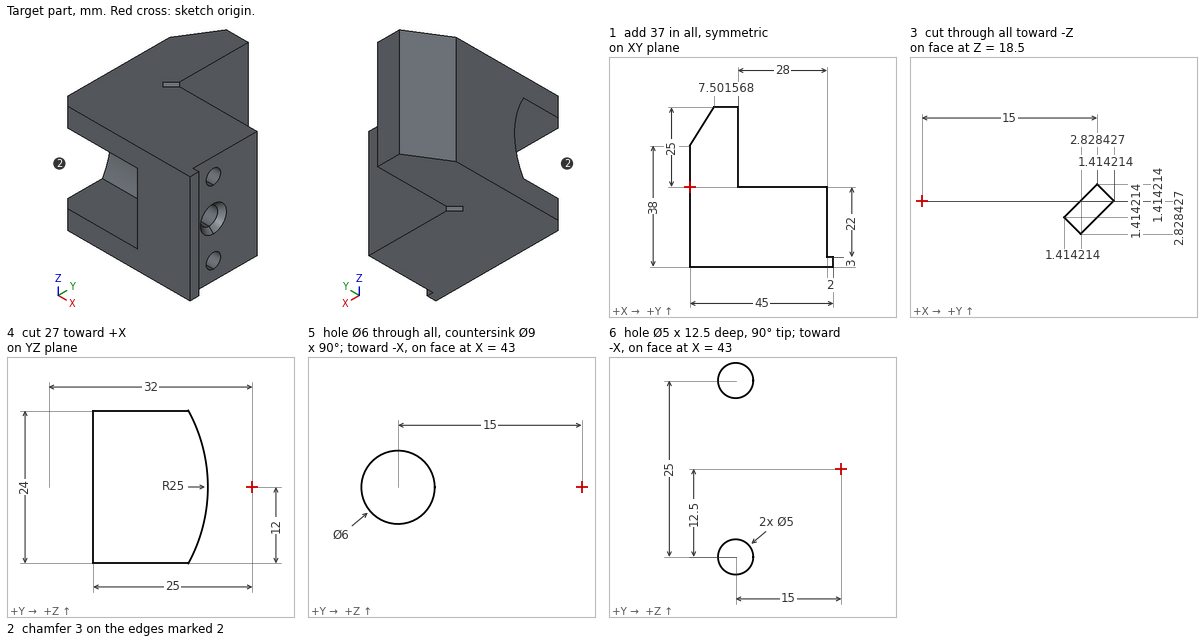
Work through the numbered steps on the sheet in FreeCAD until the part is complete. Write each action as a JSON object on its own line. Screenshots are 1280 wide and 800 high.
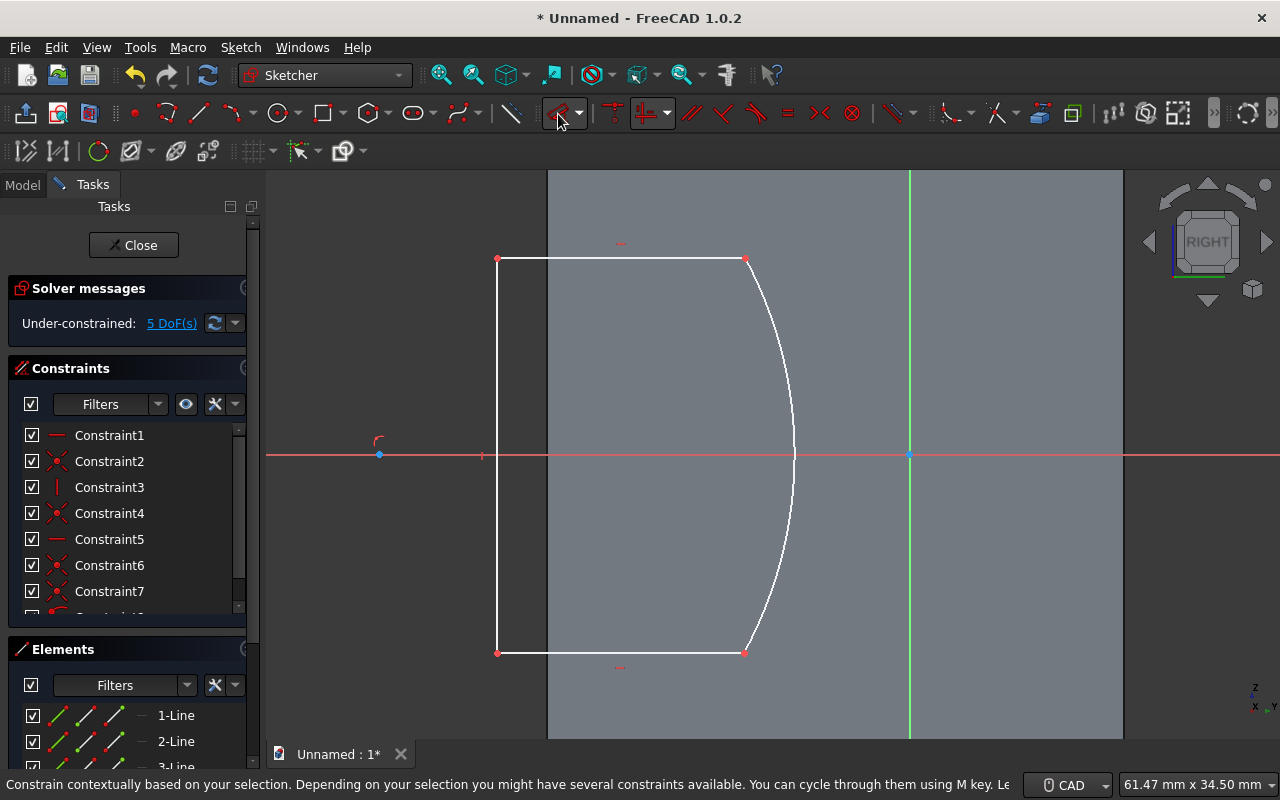
{"action": "left_click", "coordinate": [786, 537]}
{"action": "left_click", "coordinate": [817, 543]}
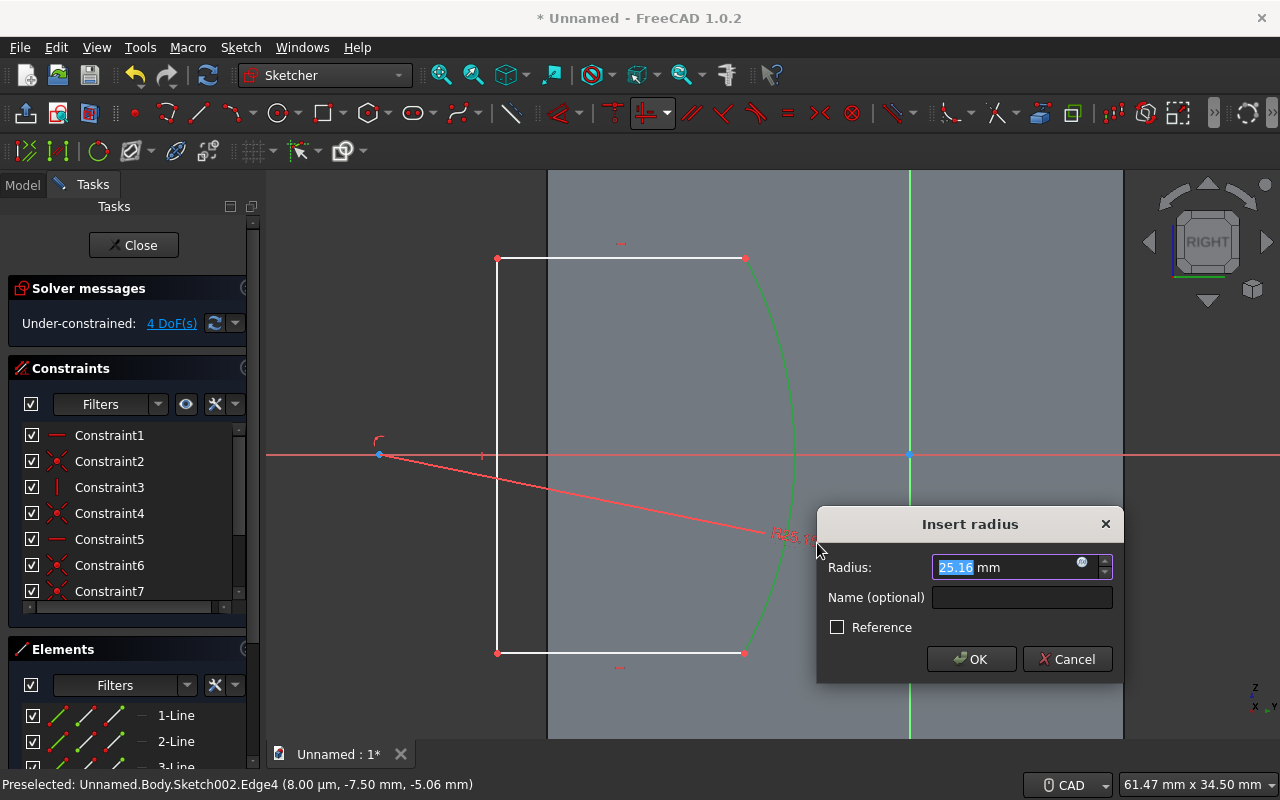
{"action": "type", "text": "25"}
{"action": "key", "text": "Return"}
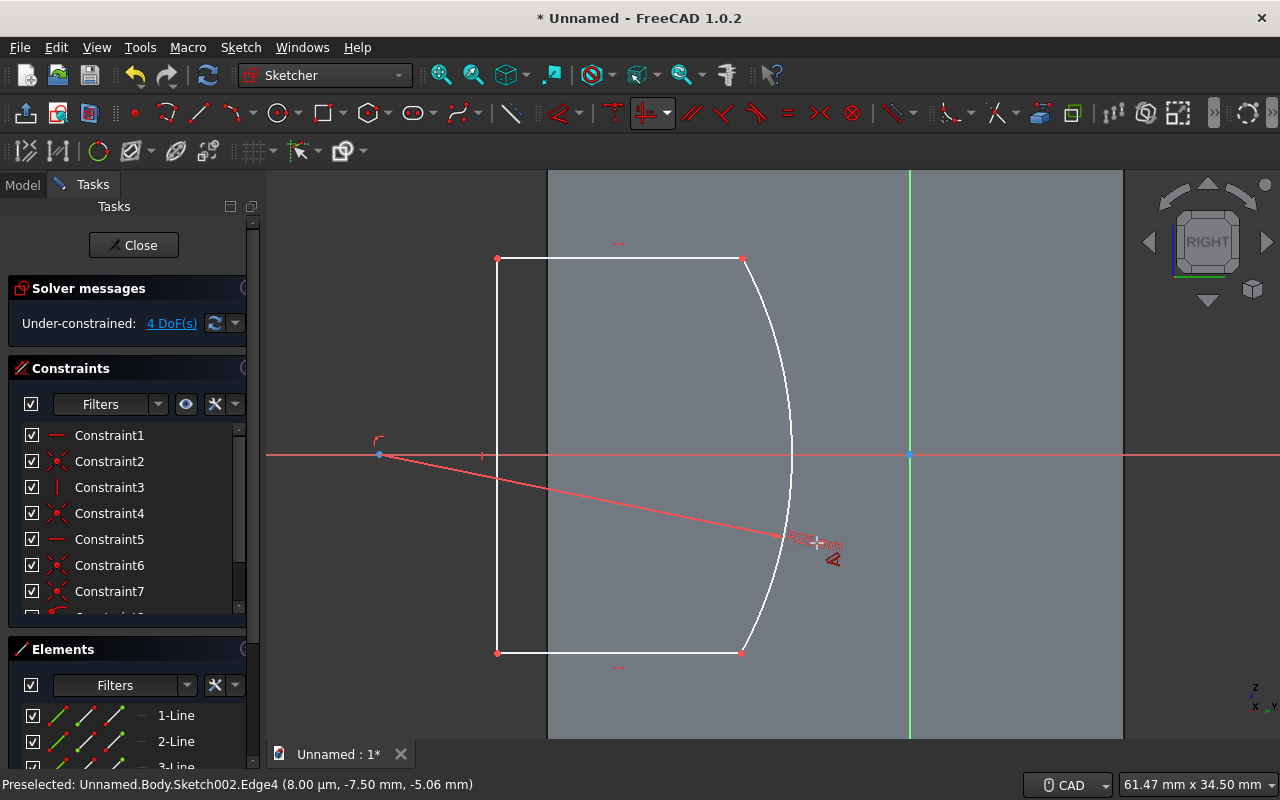
{"action": "left_click", "coordinate": [497, 535]}
{"action": "left_click", "coordinate": [463, 365]}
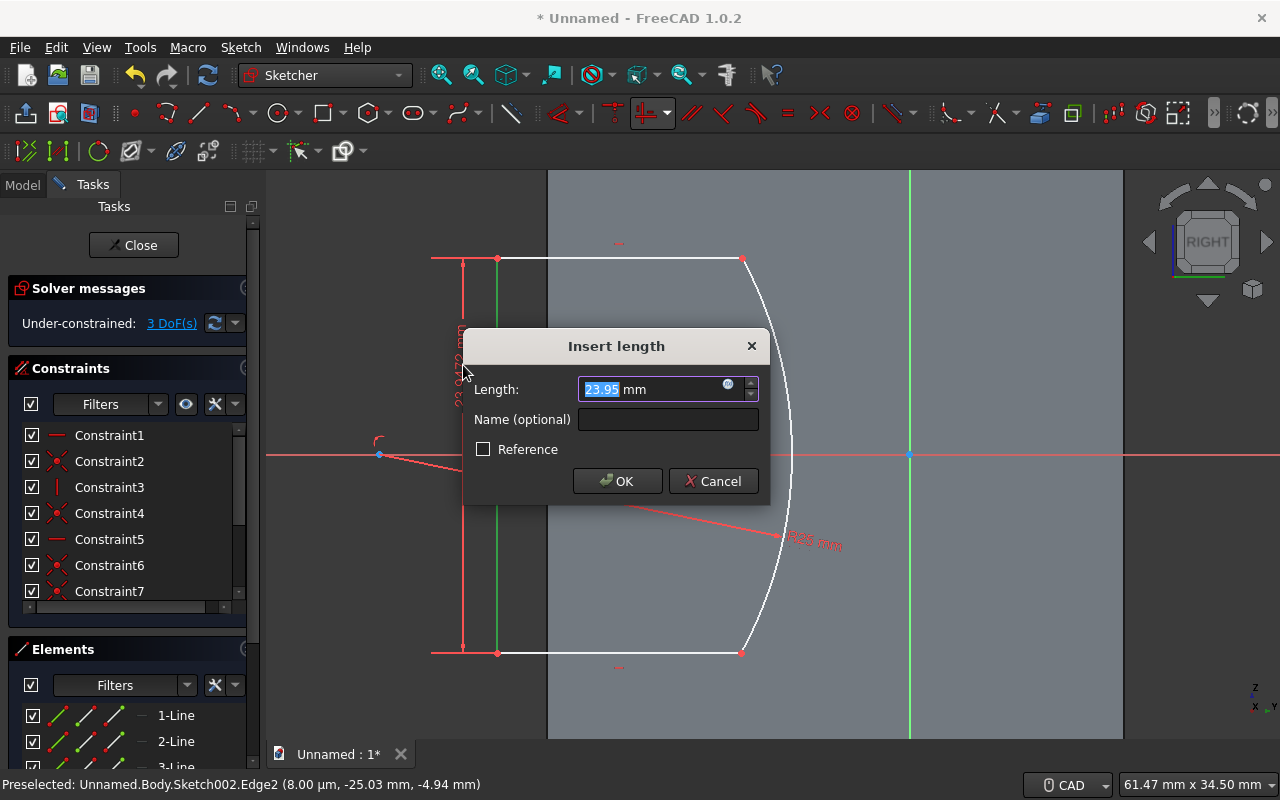
{"action": "type", "text": "24"}
{"action": "key", "text": "Return"}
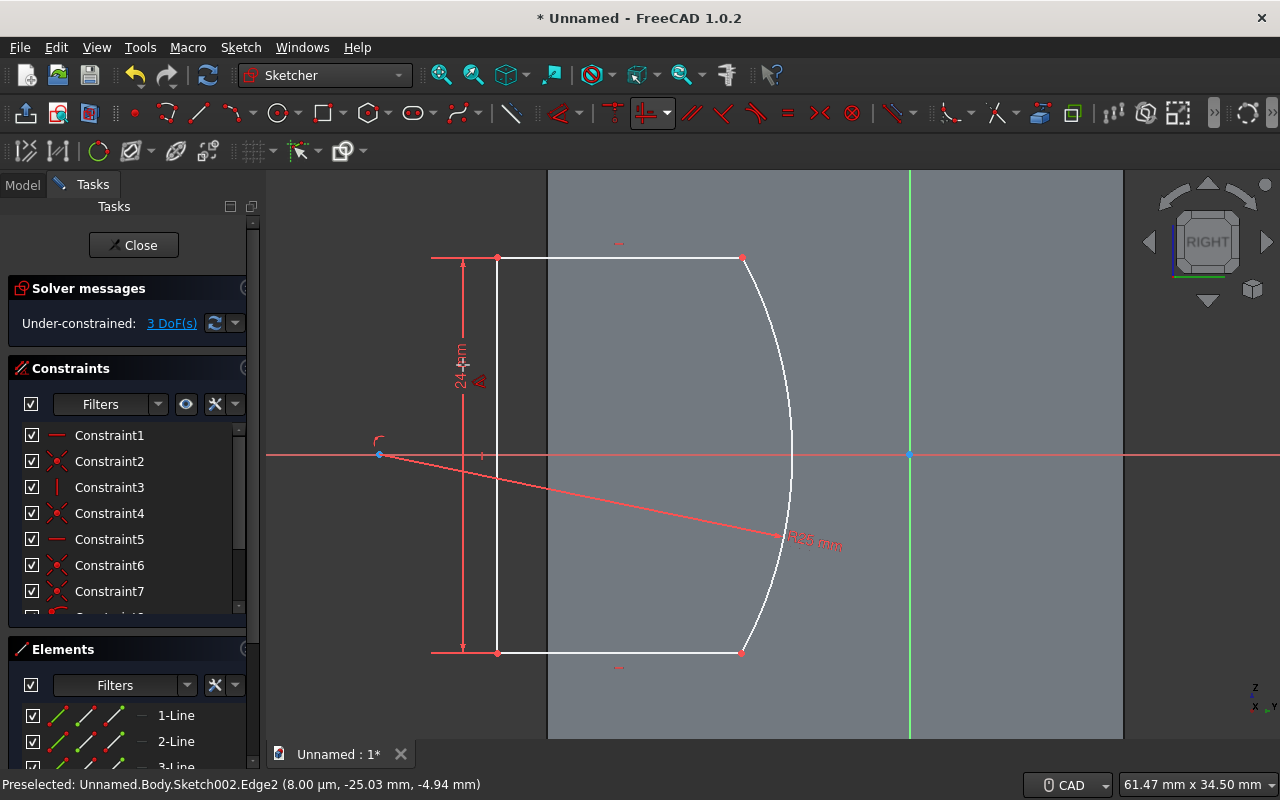
{"action": "left_click", "coordinate": [741, 653]}
{"action": "left_click", "coordinate": [944, 554]}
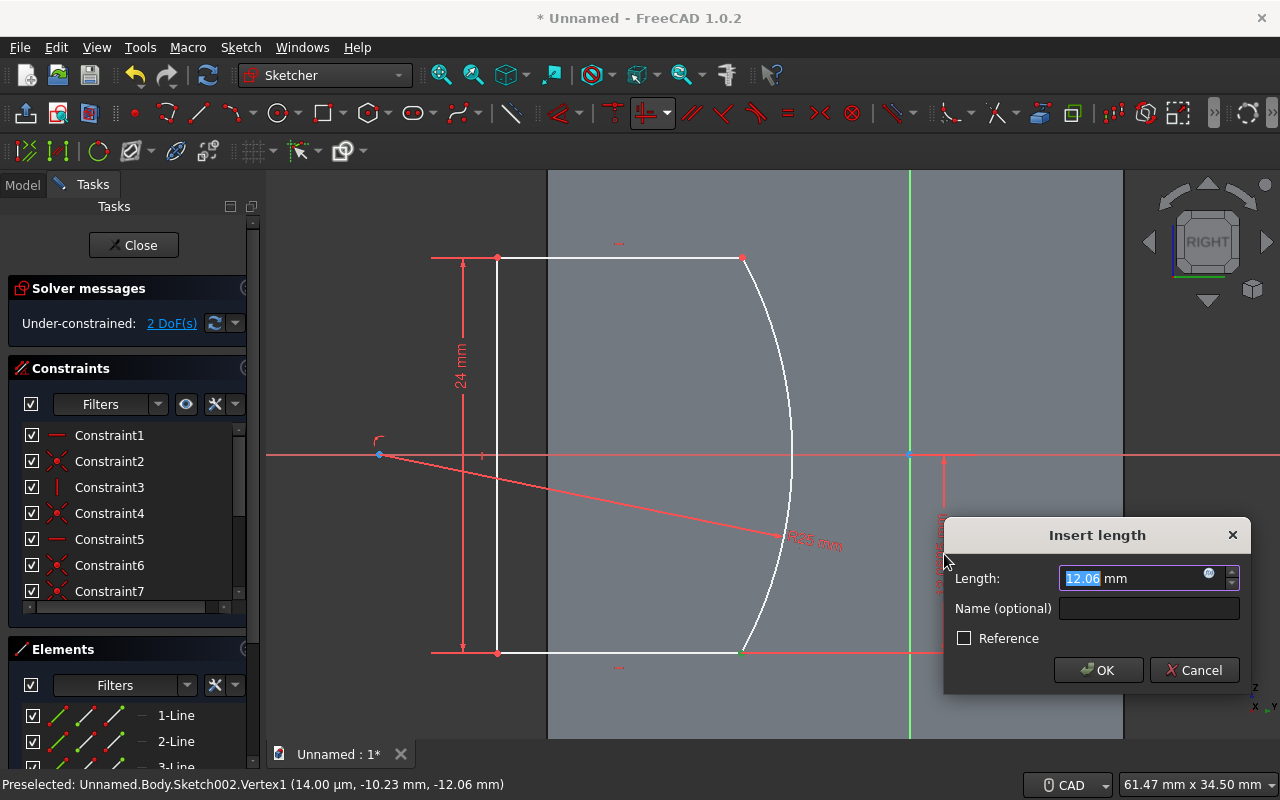
{"action": "type", "text": "12"}
{"action": "key", "text": "Return"}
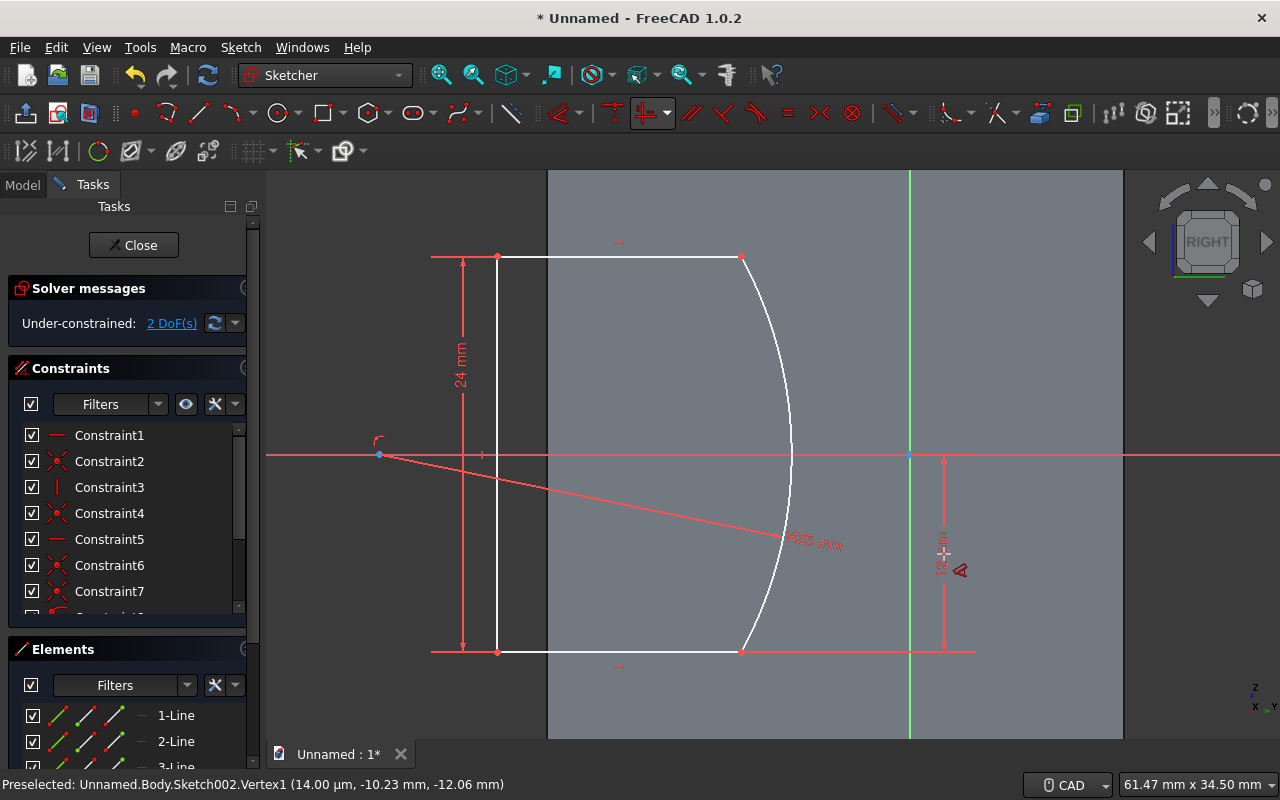
{"action": "left_click", "coordinate": [497, 652]}
{"action": "left_click", "coordinate": [703, 686]}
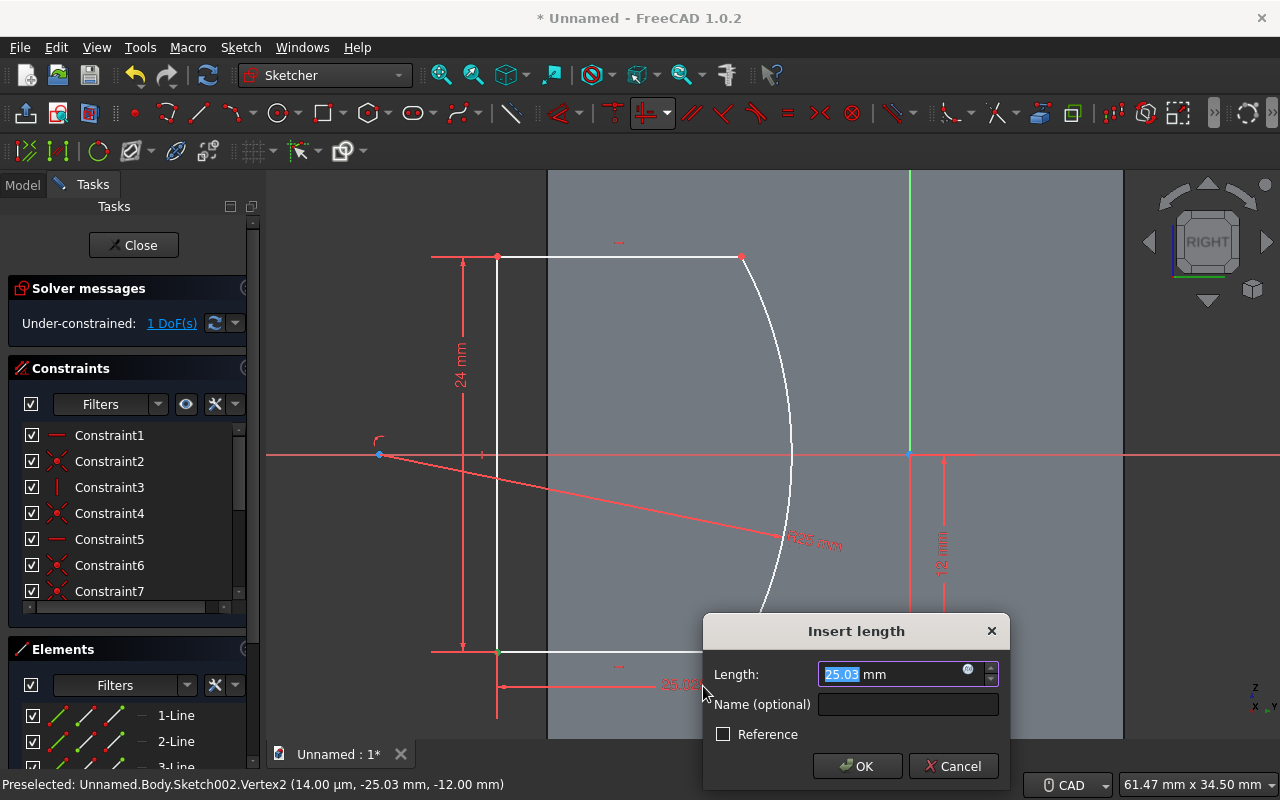
{"action": "type", "text": "25"}
{"action": "key", "text": "Return"}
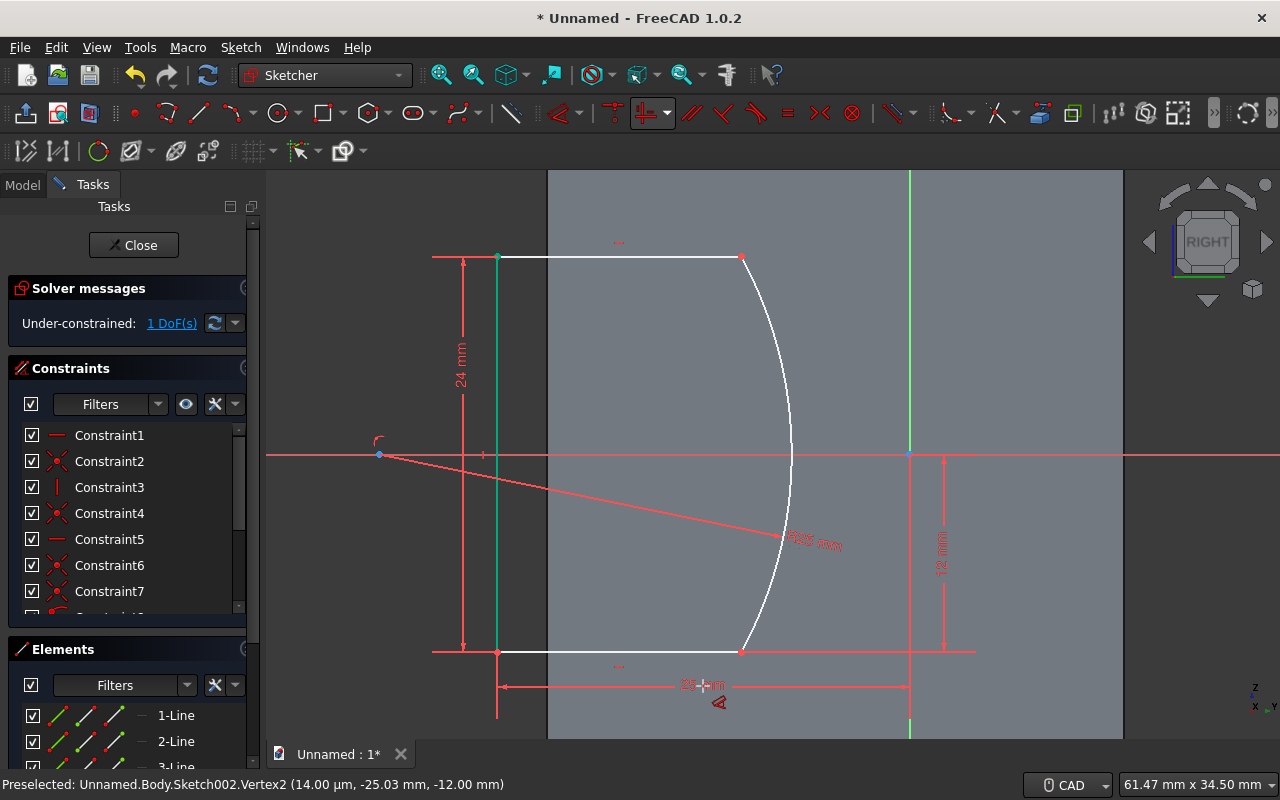
{"action": "left_click", "coordinate": [379, 454]}
{"action": "left_click", "coordinate": [645, 488]}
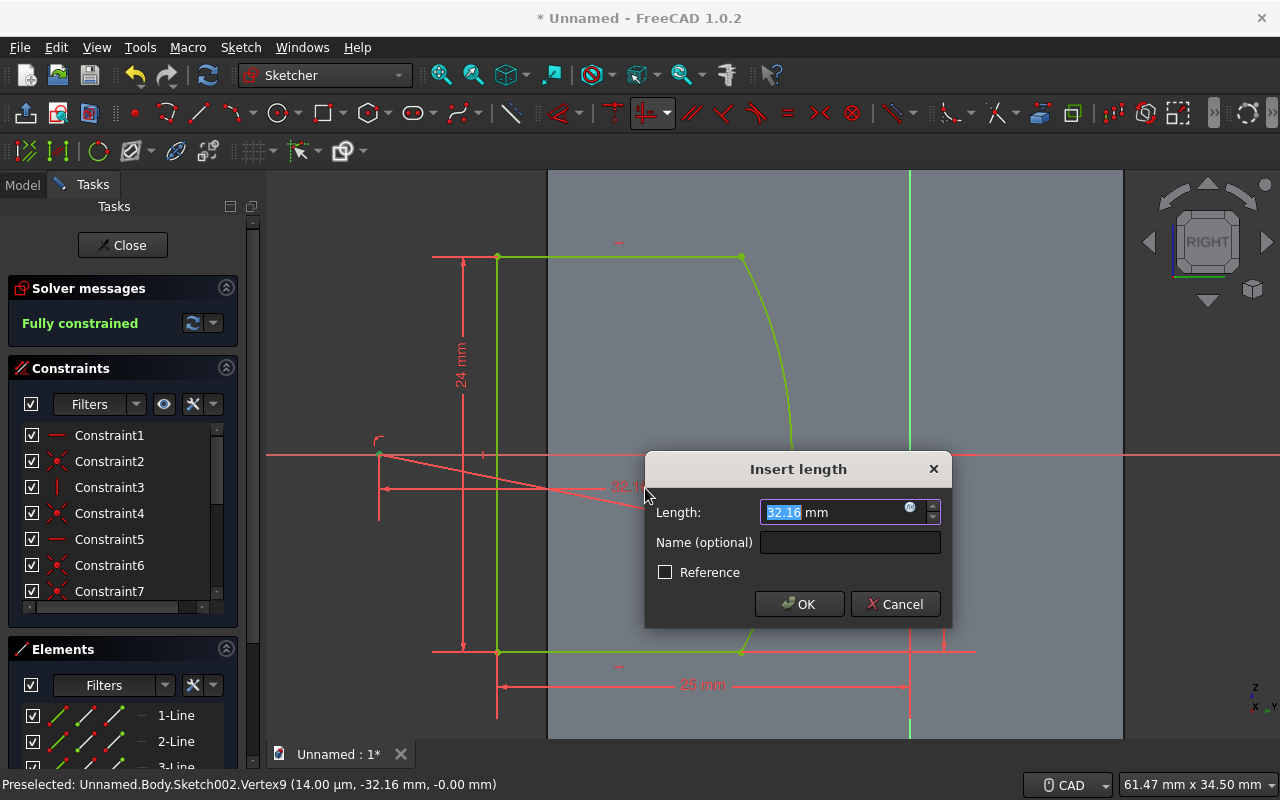
{"action": "type", "text": "32"}
{"action": "key", "text": "Return"}
{"action": "key", "text": "Escape"}